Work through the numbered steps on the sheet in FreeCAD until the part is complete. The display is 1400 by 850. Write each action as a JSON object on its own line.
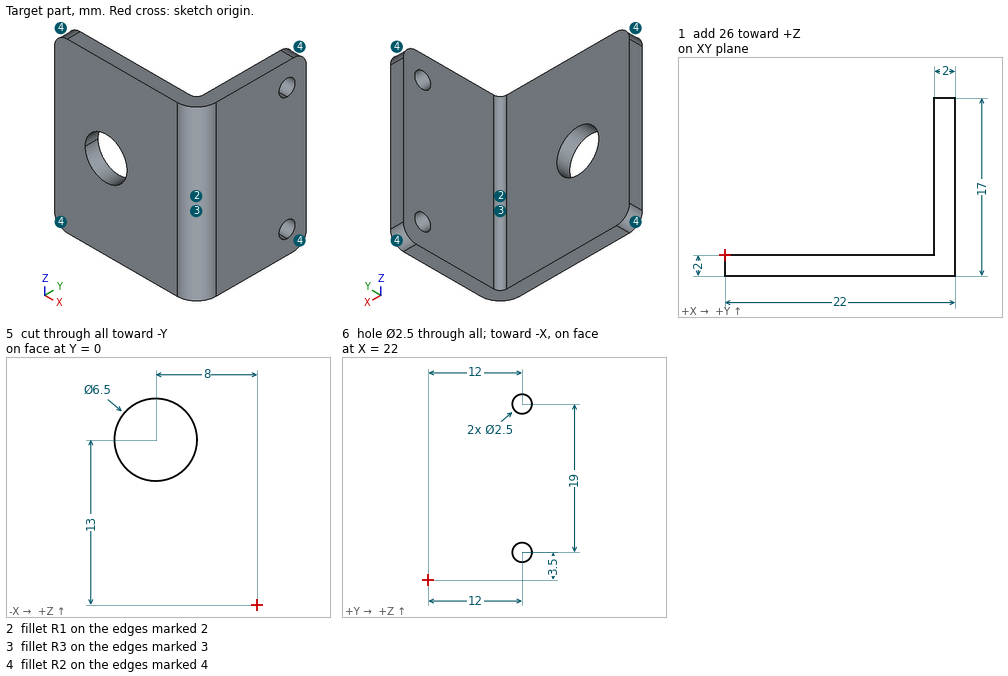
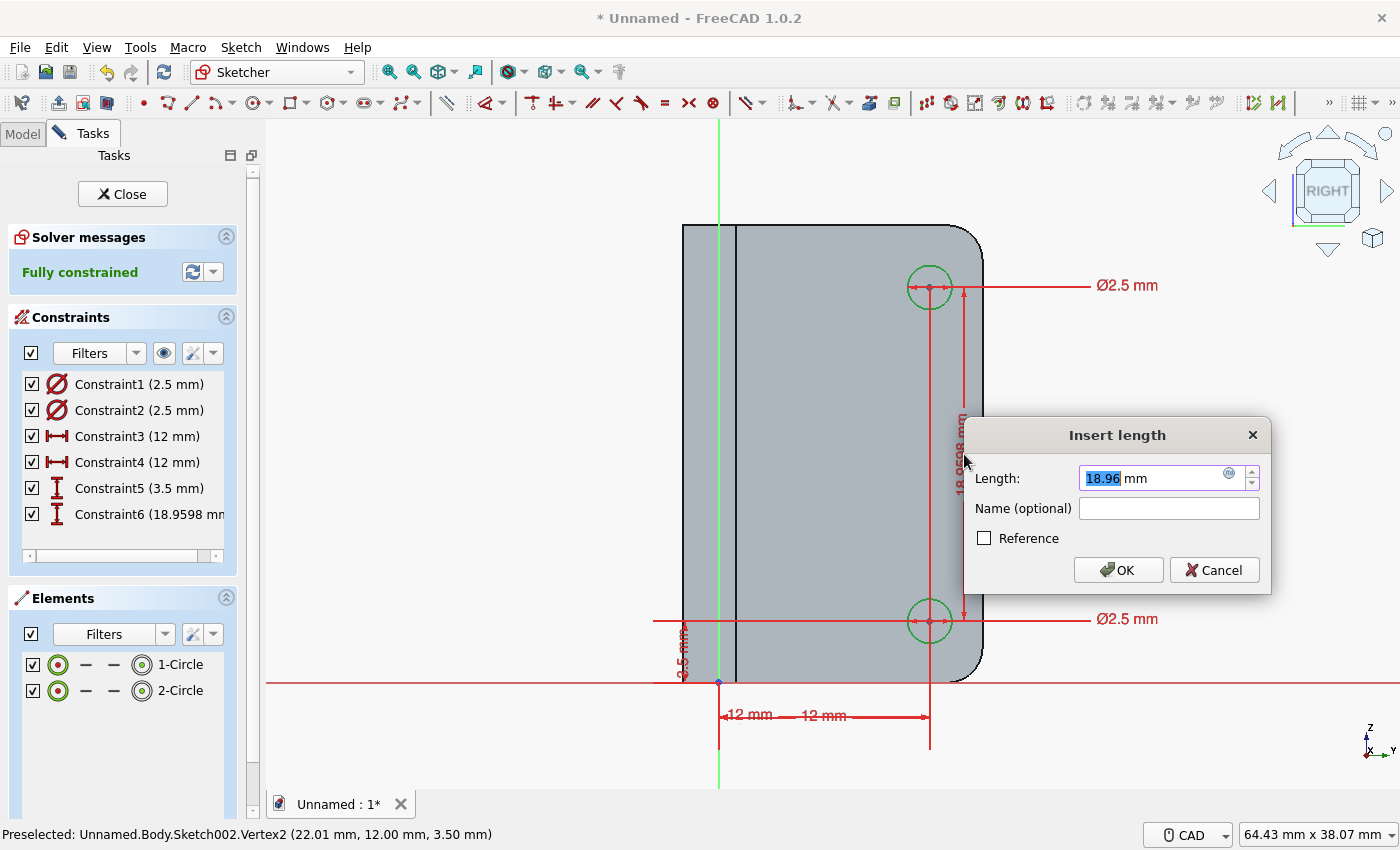
{"action": "type", "text": "19"}
{"action": "key", "text": "Return"}
{"action": "key", "text": "Escape"}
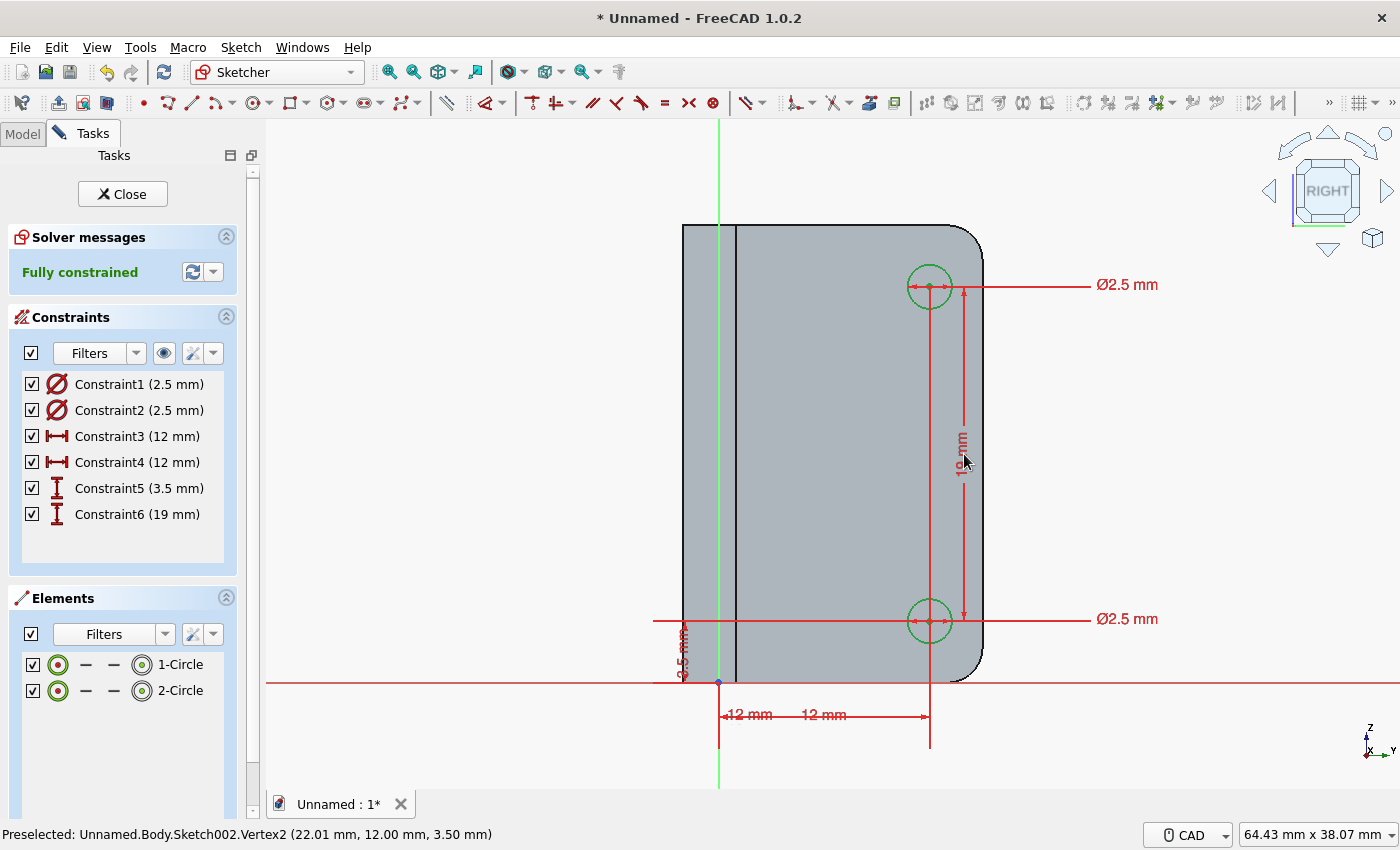
{"action": "left_click", "coordinate": [123, 194]}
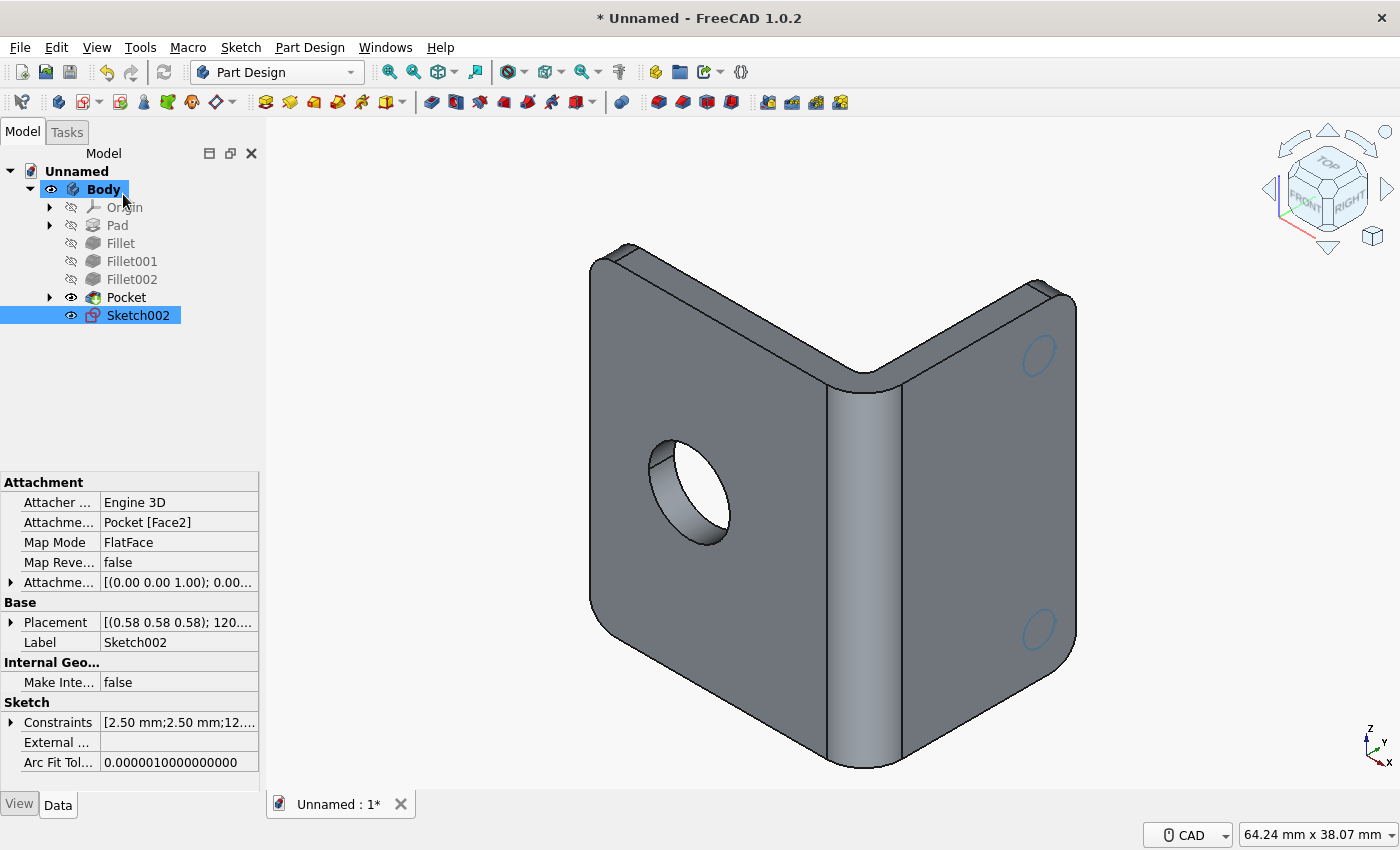
{"action": "left_click", "coordinate": [456, 102]}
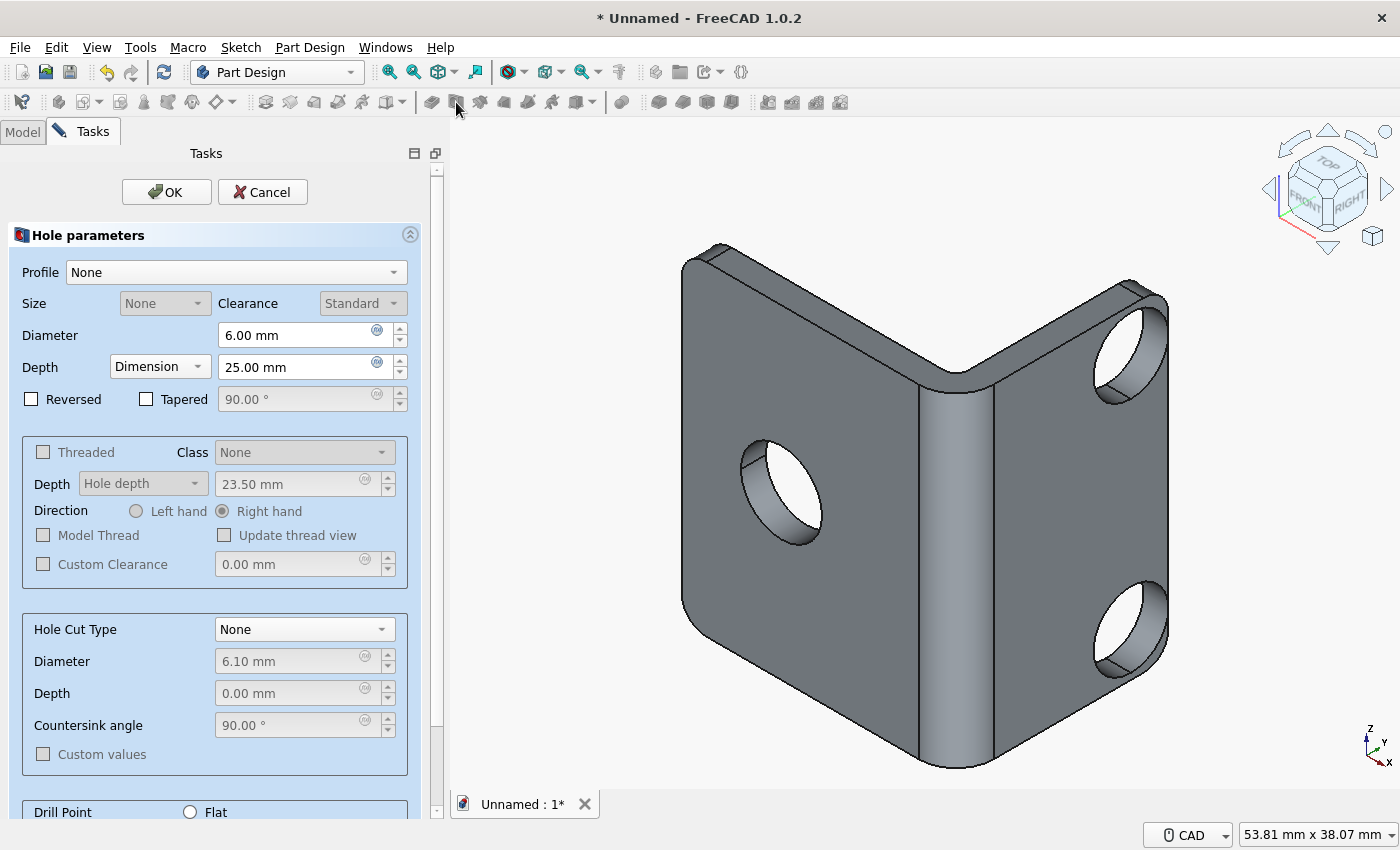
{"action": "triple_click", "coordinate": [305, 335]}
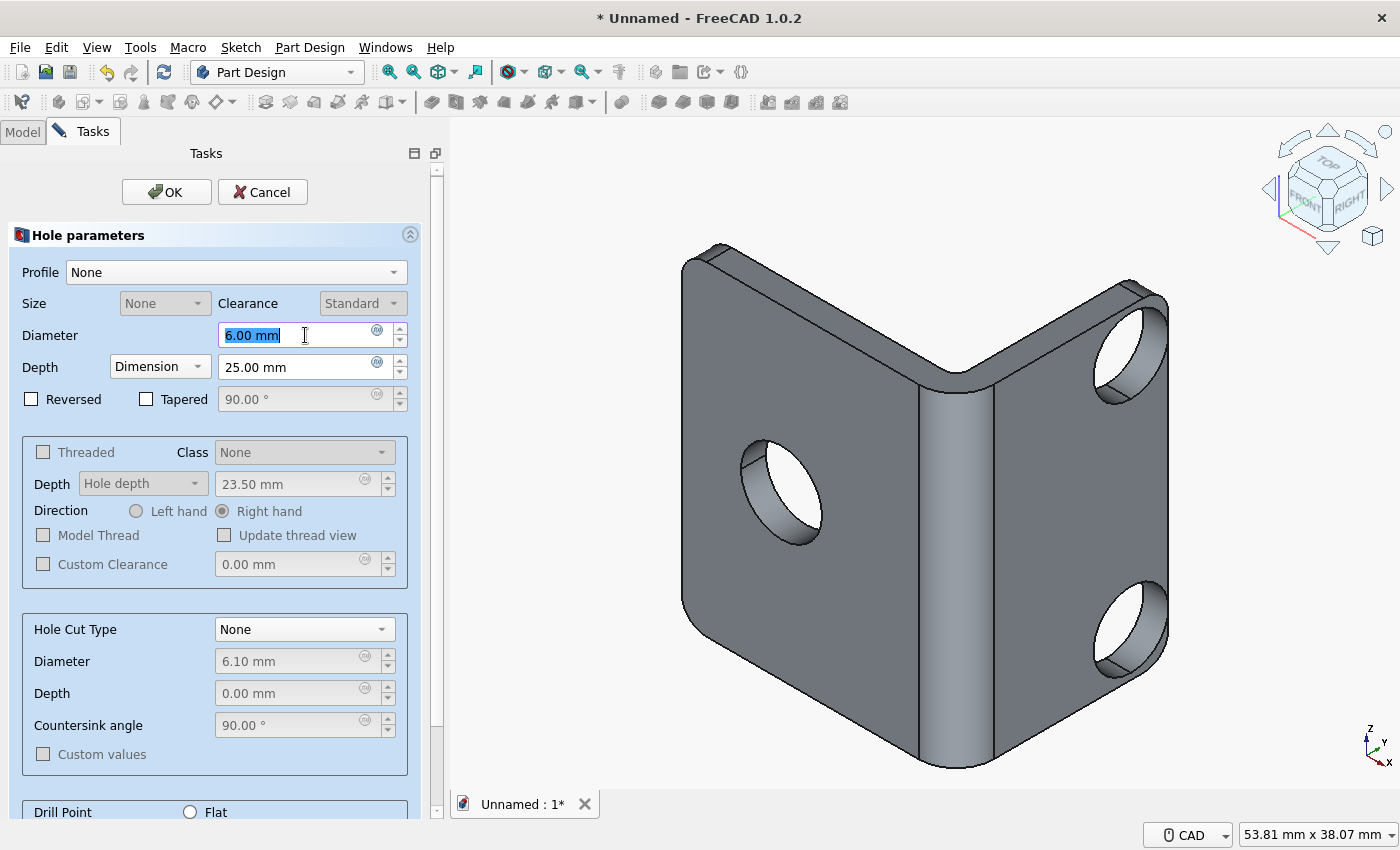
{"action": "type", "text": "2.5"}
{"action": "key", "text": "Tab"}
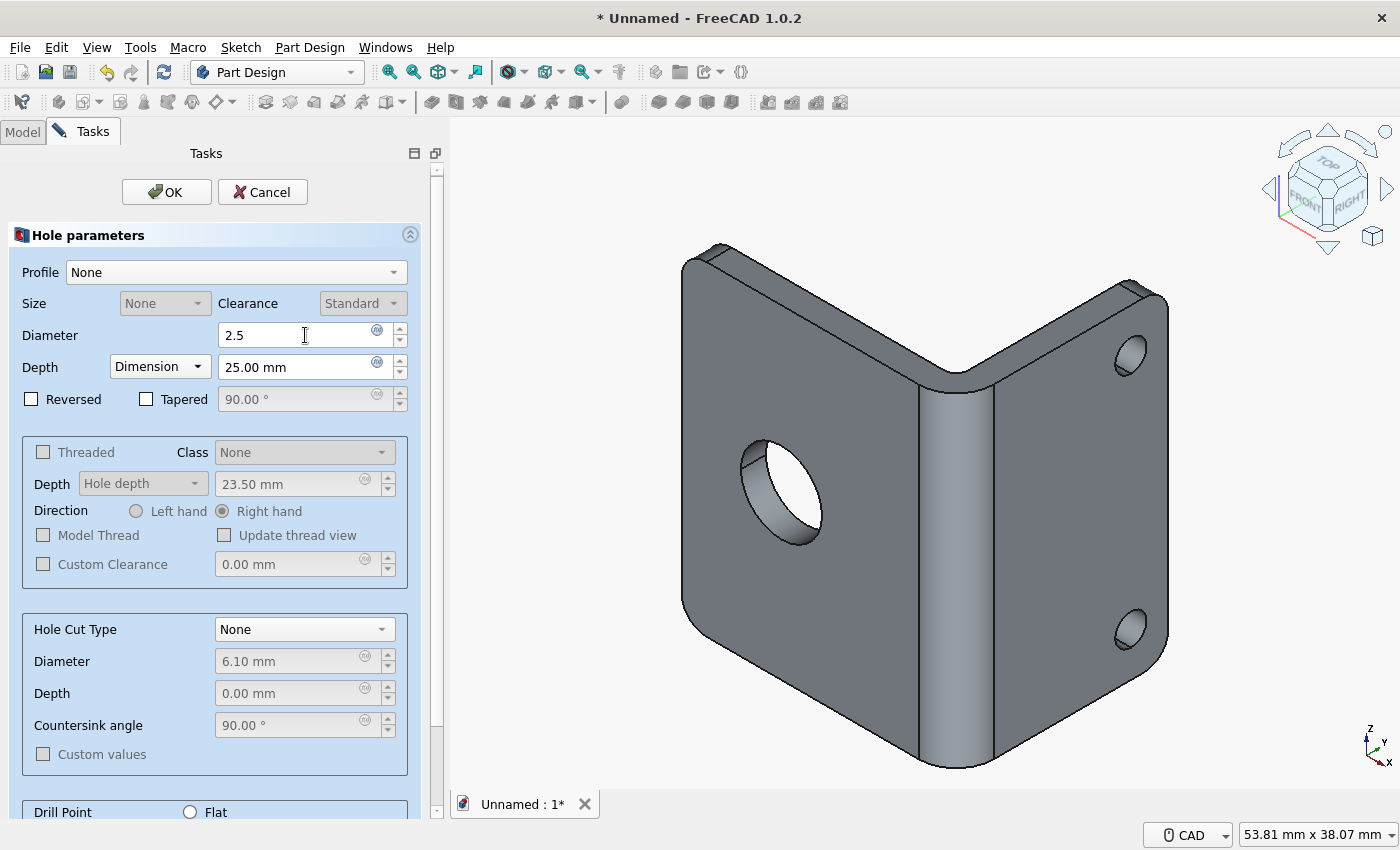
{"action": "left_click", "coordinate": [161, 366]}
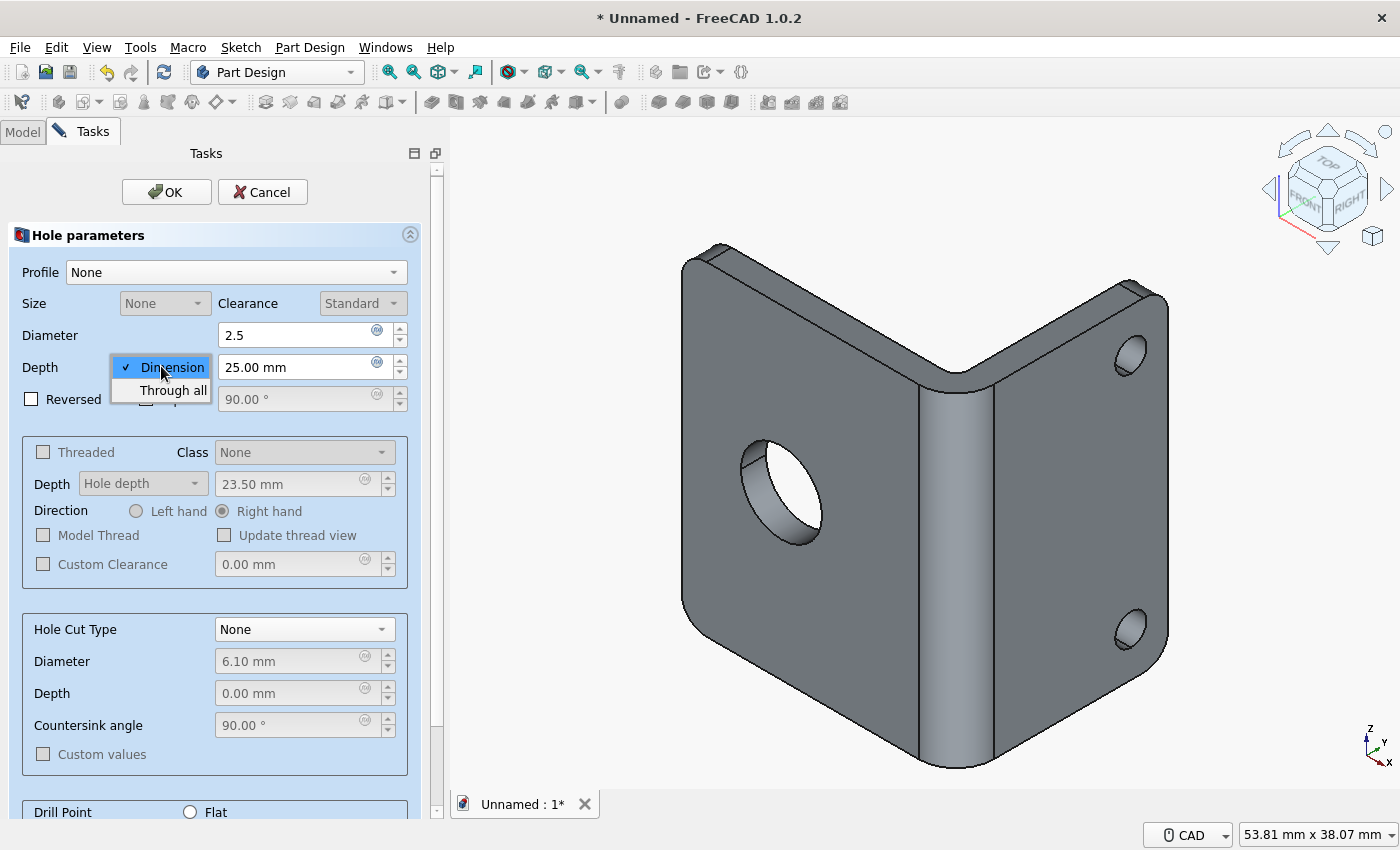
{"action": "left_click", "coordinate": [160, 390]}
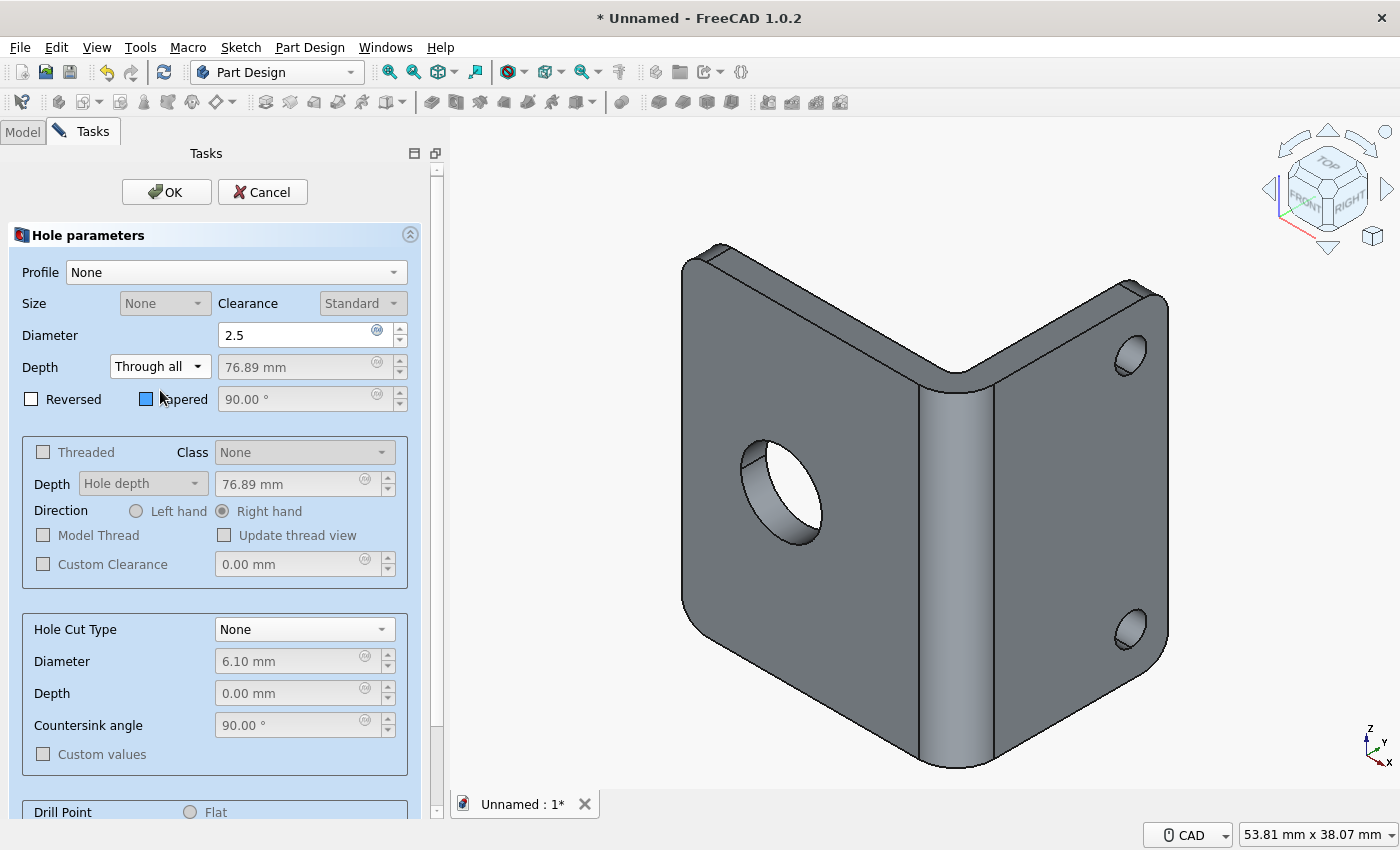
{"action": "left_click", "coordinate": [167, 192]}